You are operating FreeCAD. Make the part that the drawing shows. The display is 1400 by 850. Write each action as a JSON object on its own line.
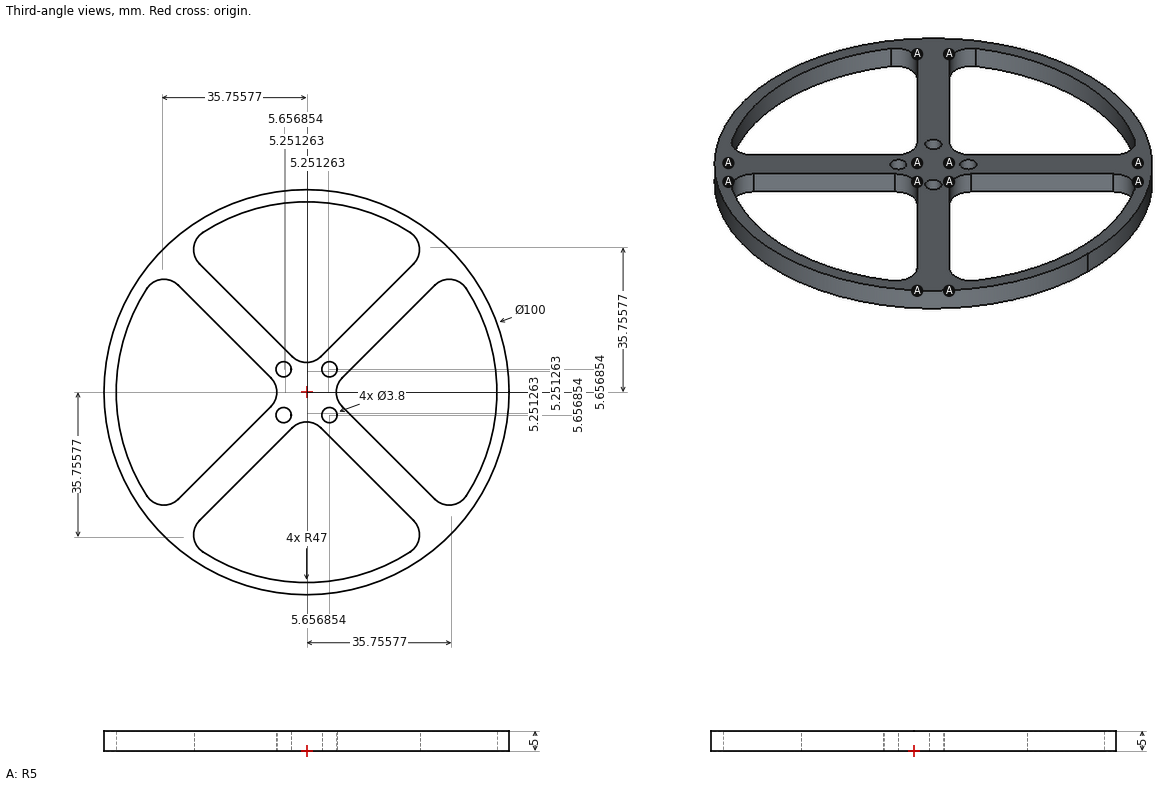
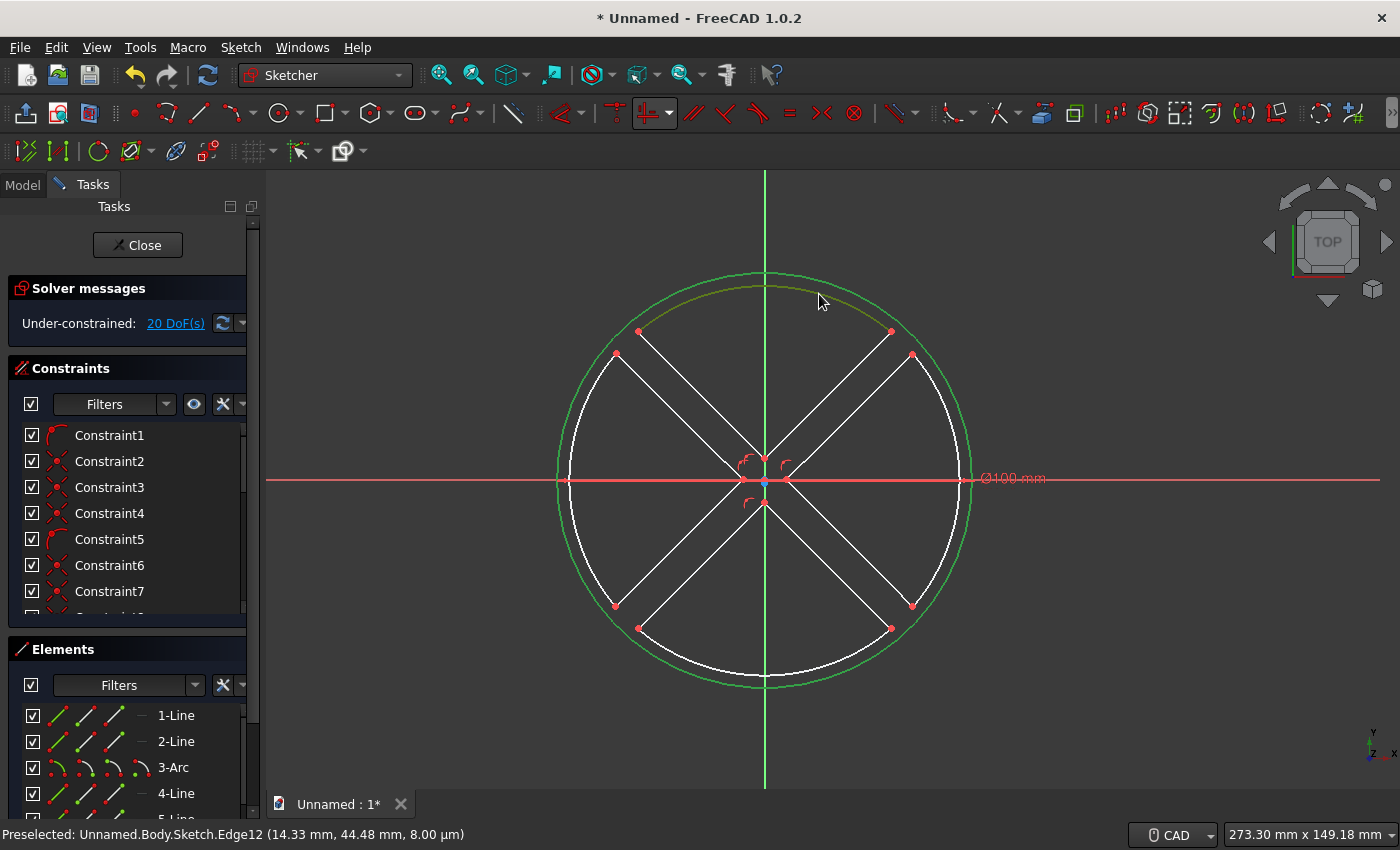
{"action": "left_click", "coordinate": [616, 114]}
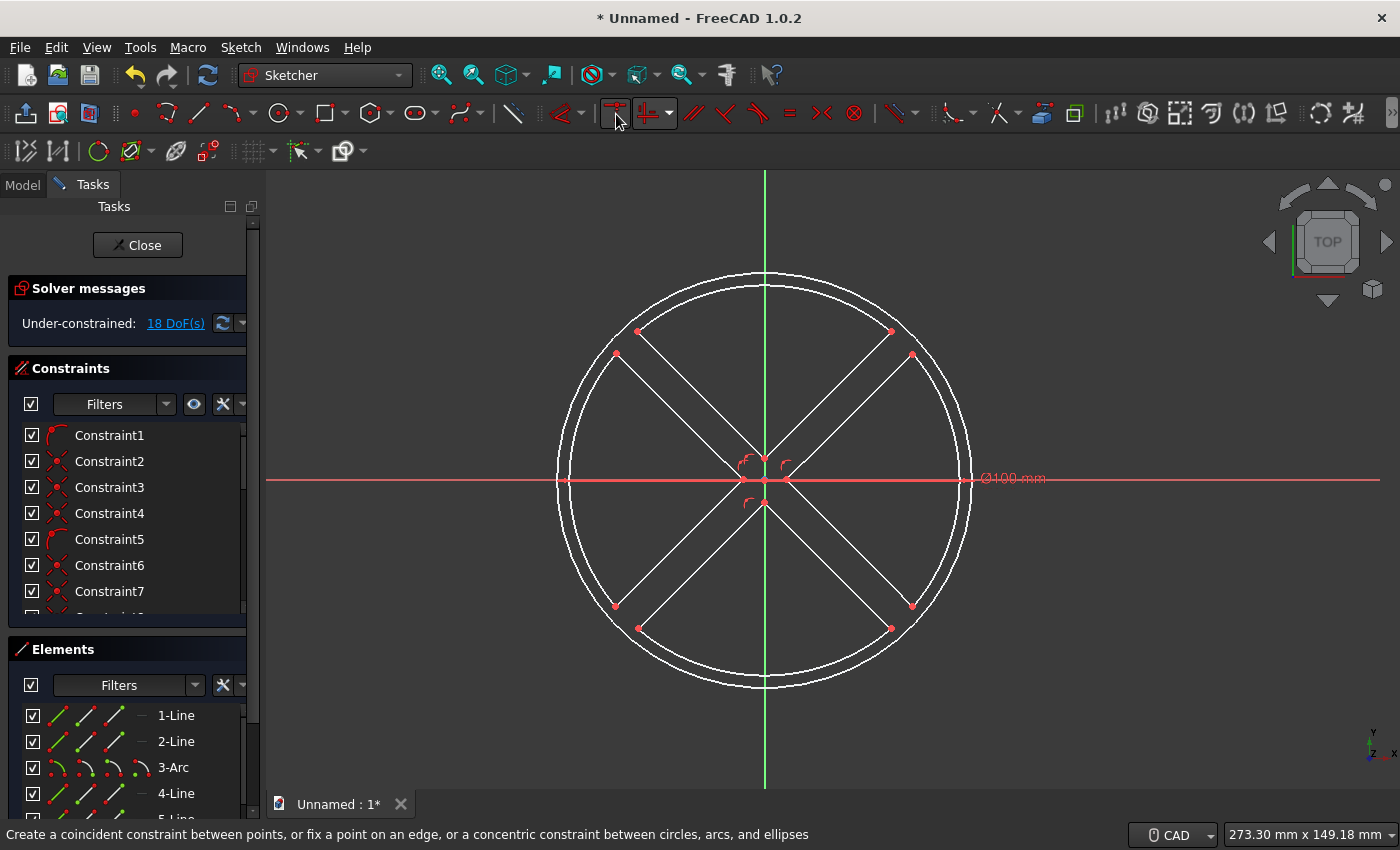
{"action": "scroll", "coordinate": [765, 480], "scroll_direction": "up", "scroll_amount": 4}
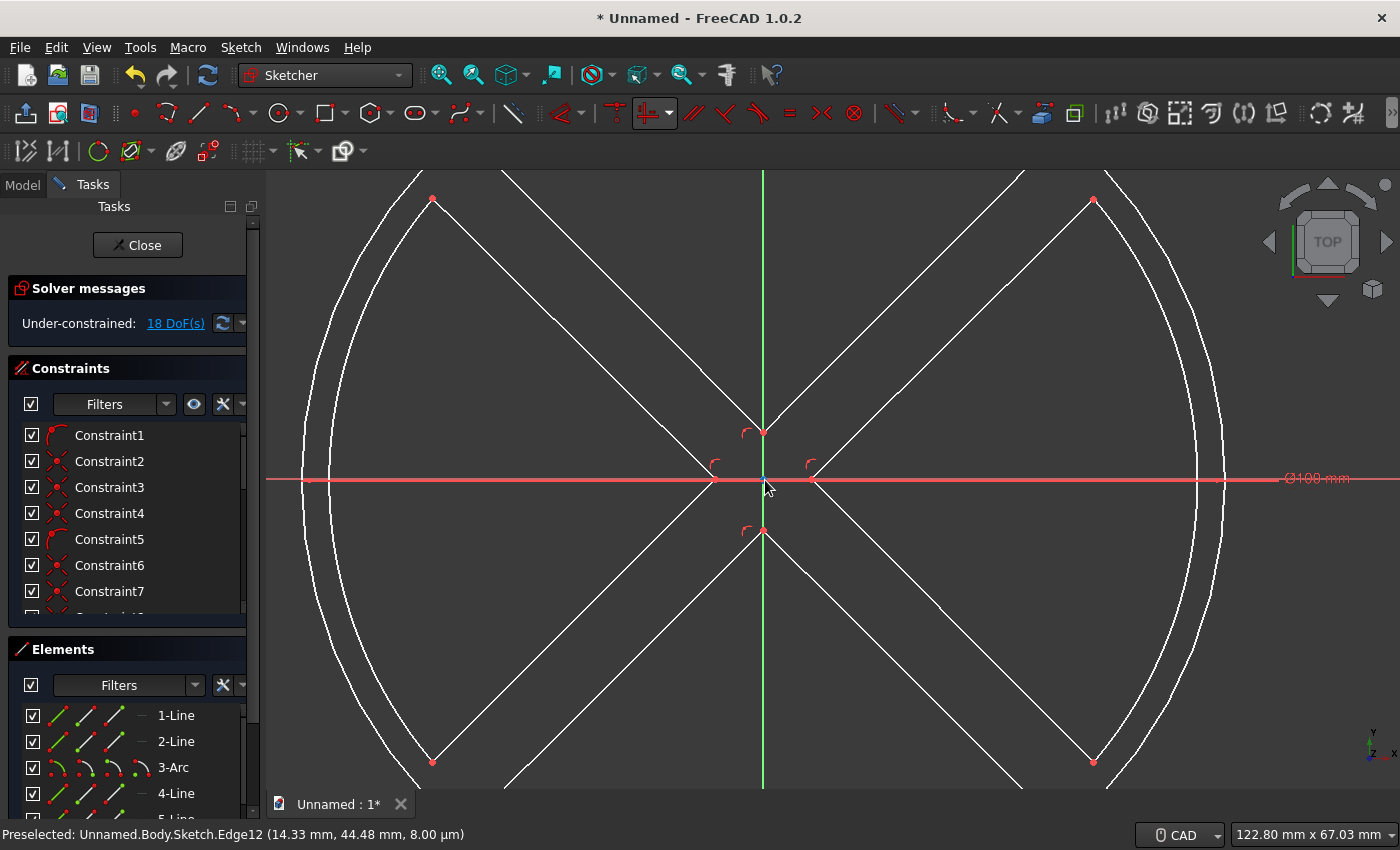
{"action": "left_click_drag", "start_coordinate": [753, 469], "coordinate": [773, 491]}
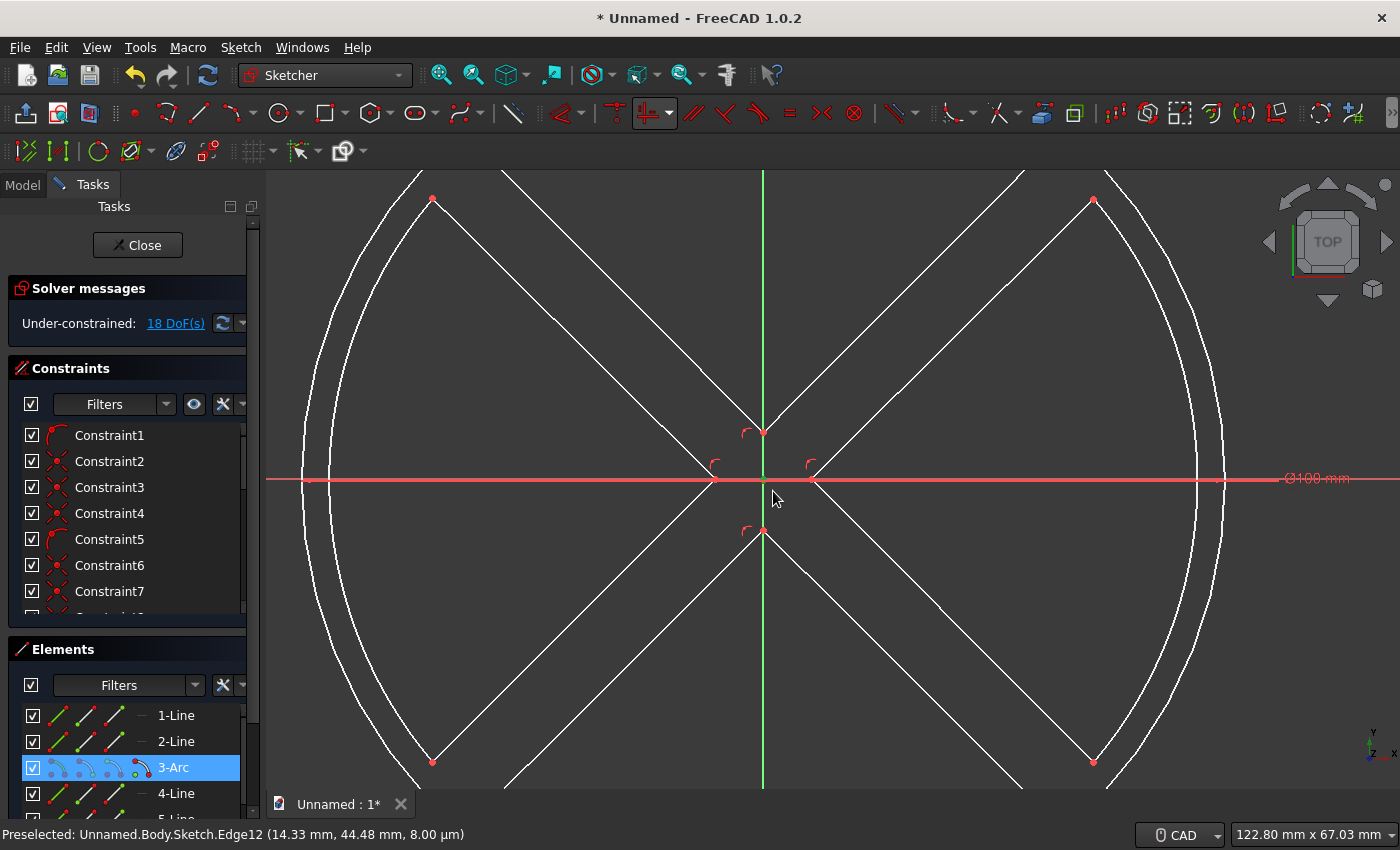
{"action": "left_click", "coordinate": [616, 114]}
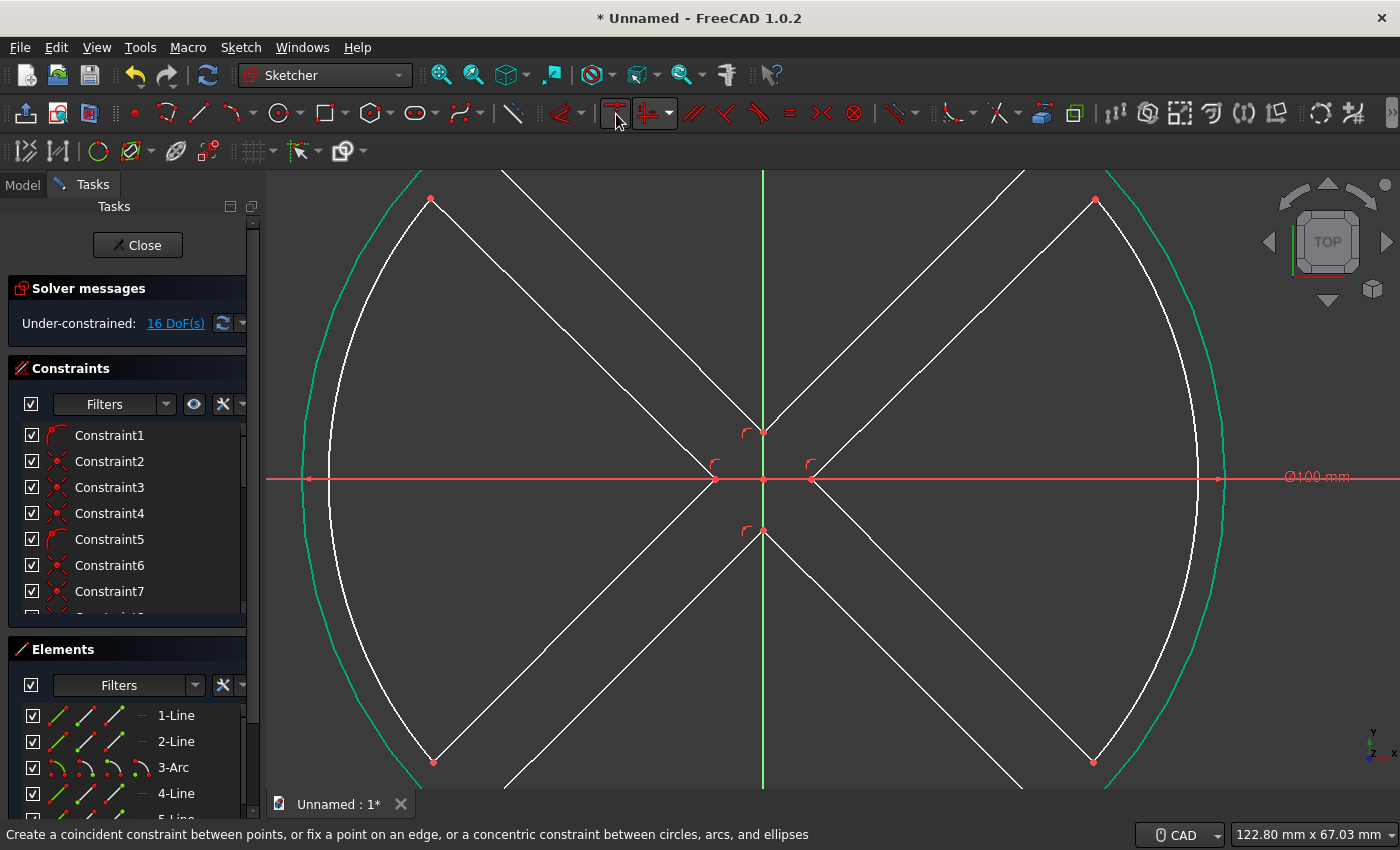
{"action": "scroll", "coordinate": [765, 480], "scroll_direction": "down", "scroll_amount": 4}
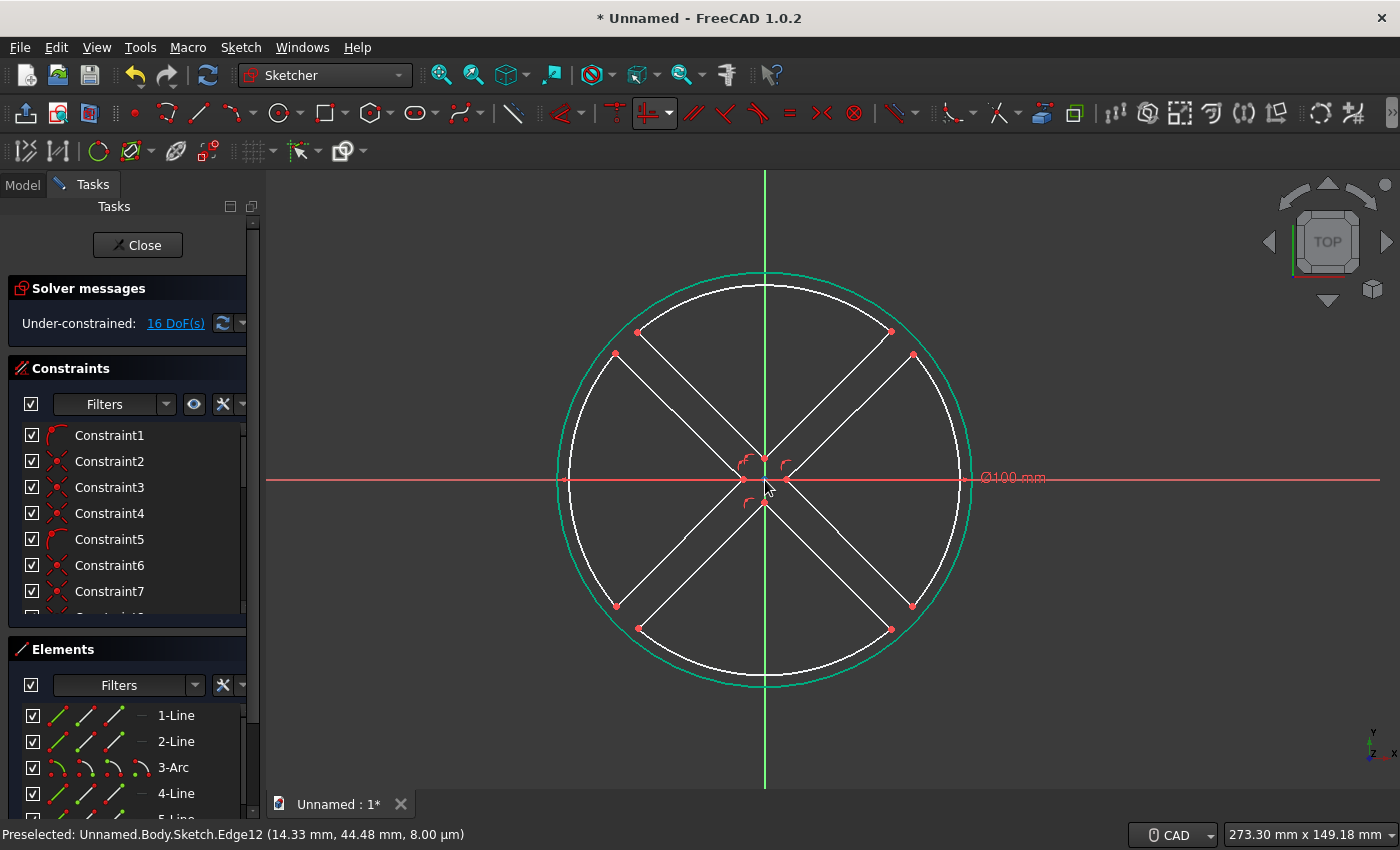
{"action": "left_click", "coordinate": [710, 668]}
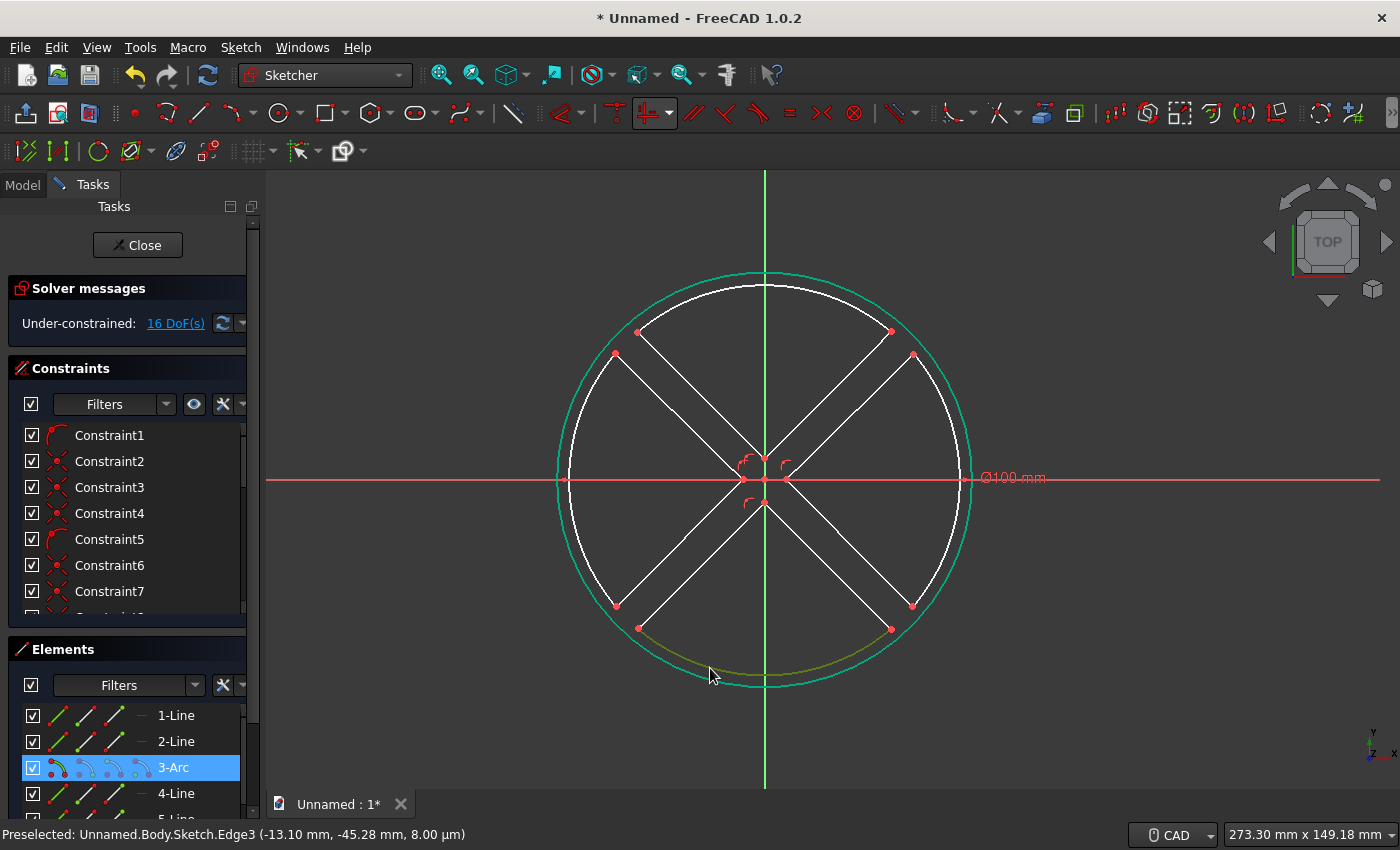
{"action": "left_click", "coordinate": [952, 535]}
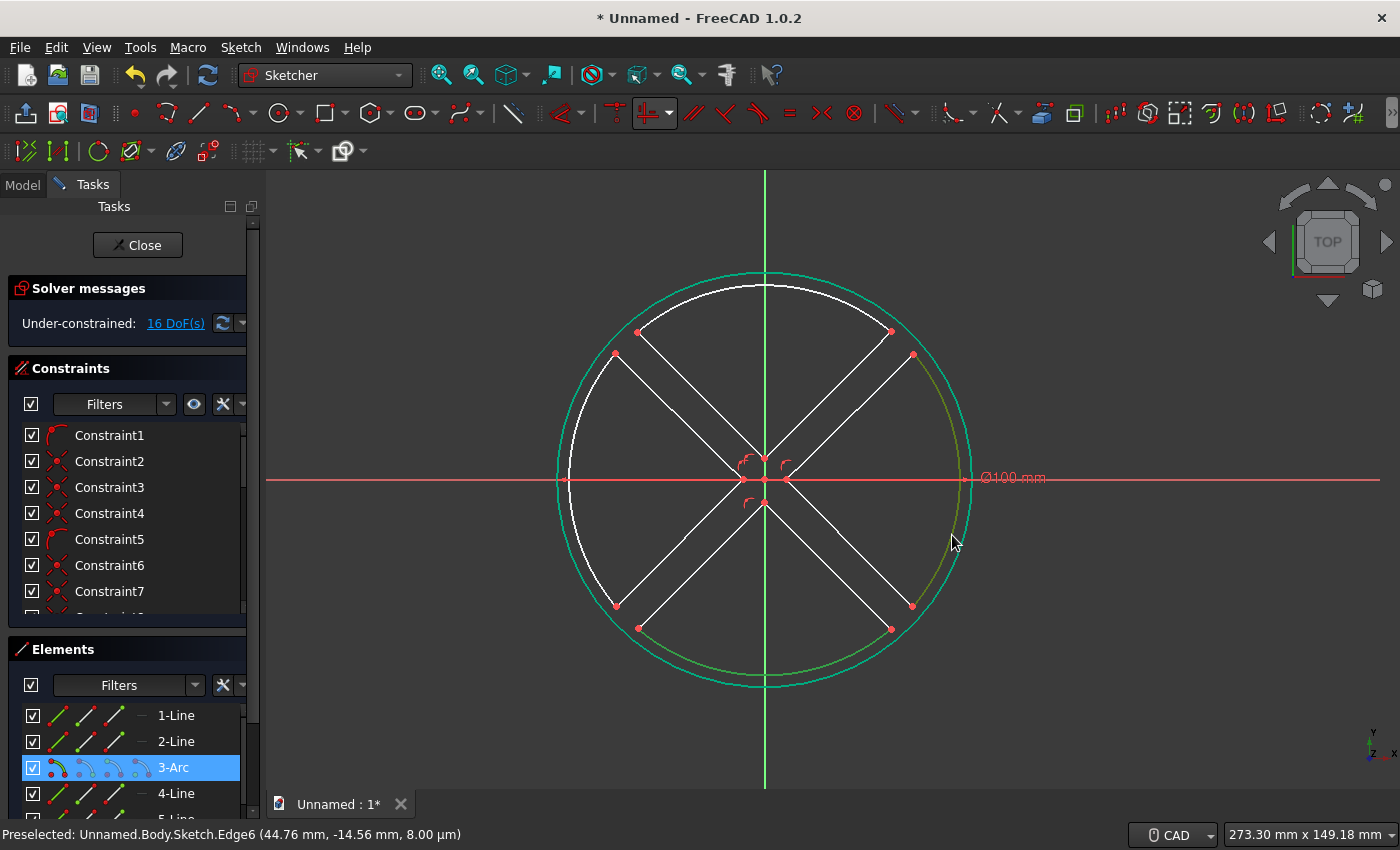
{"action": "left_click", "coordinate": [577, 426]}